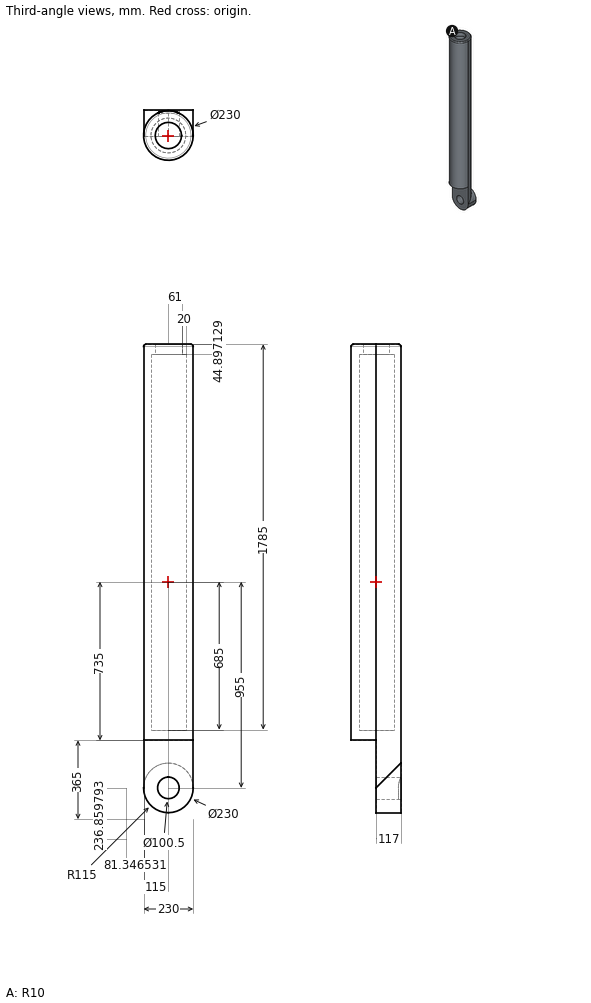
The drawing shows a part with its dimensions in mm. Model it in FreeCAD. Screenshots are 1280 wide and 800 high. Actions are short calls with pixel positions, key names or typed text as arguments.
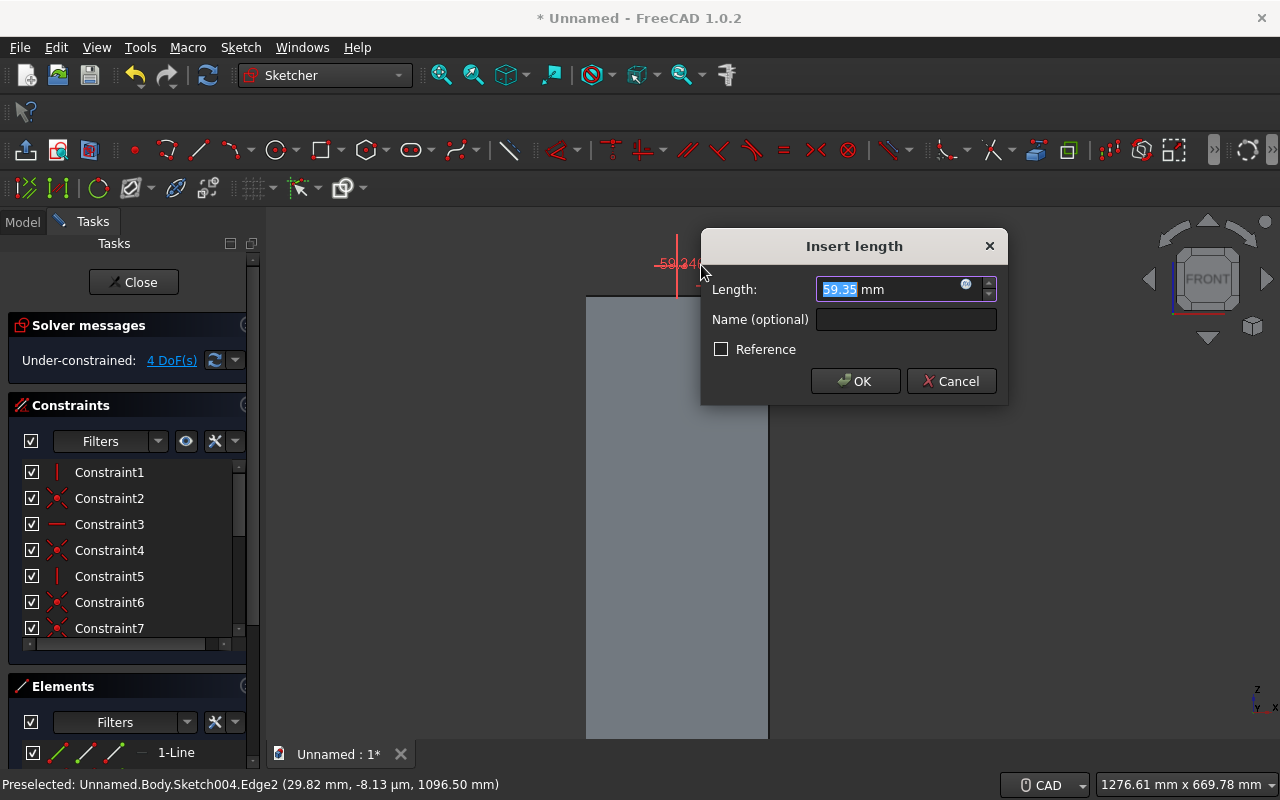
text(61)
key(Return)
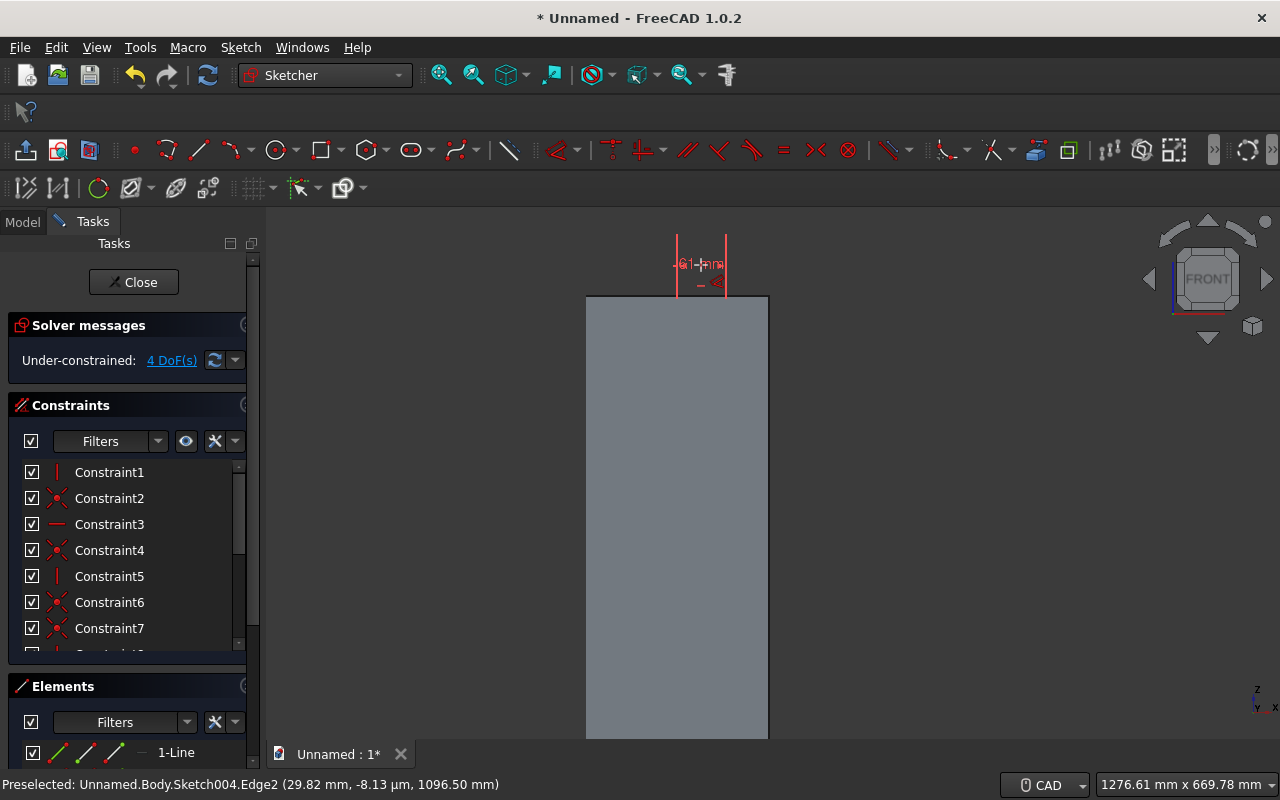
scroll(734, 336, up, 5)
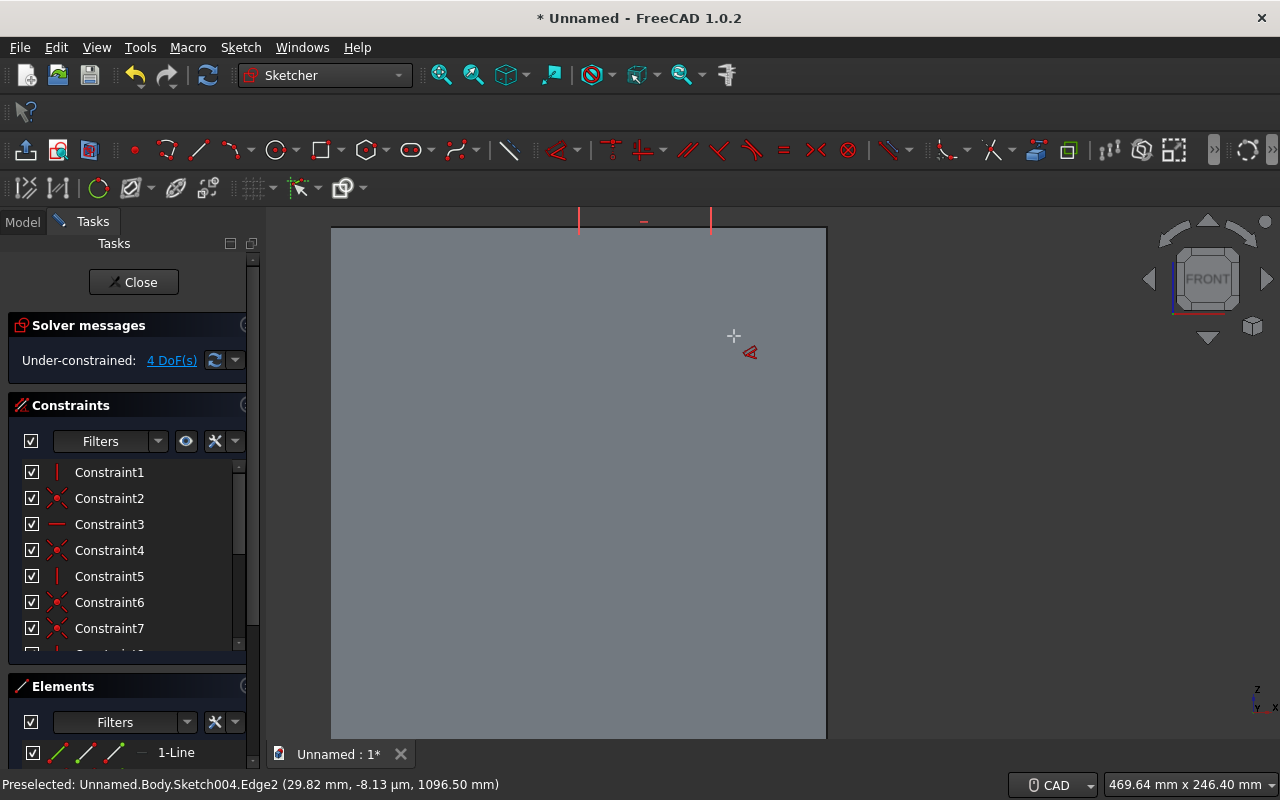
click(732, 335)
click(732, 301)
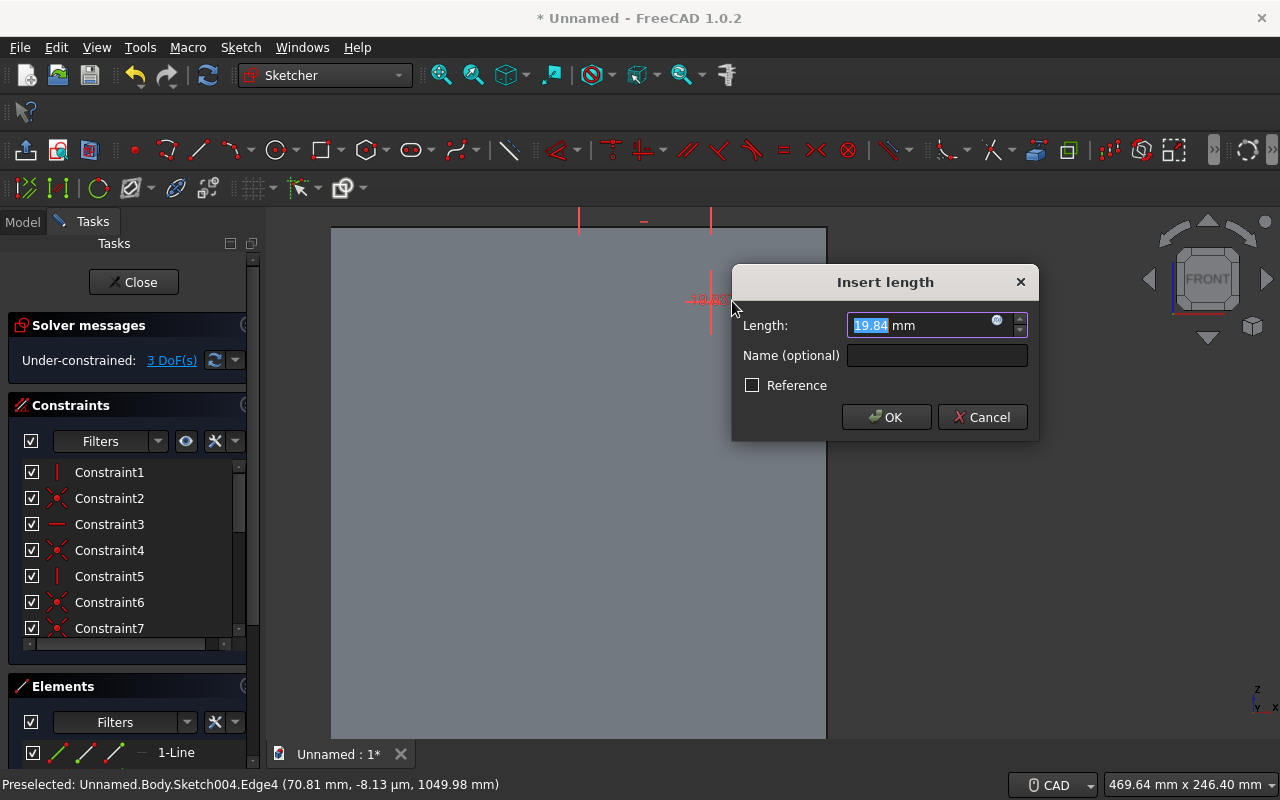
text(20)
key(Return)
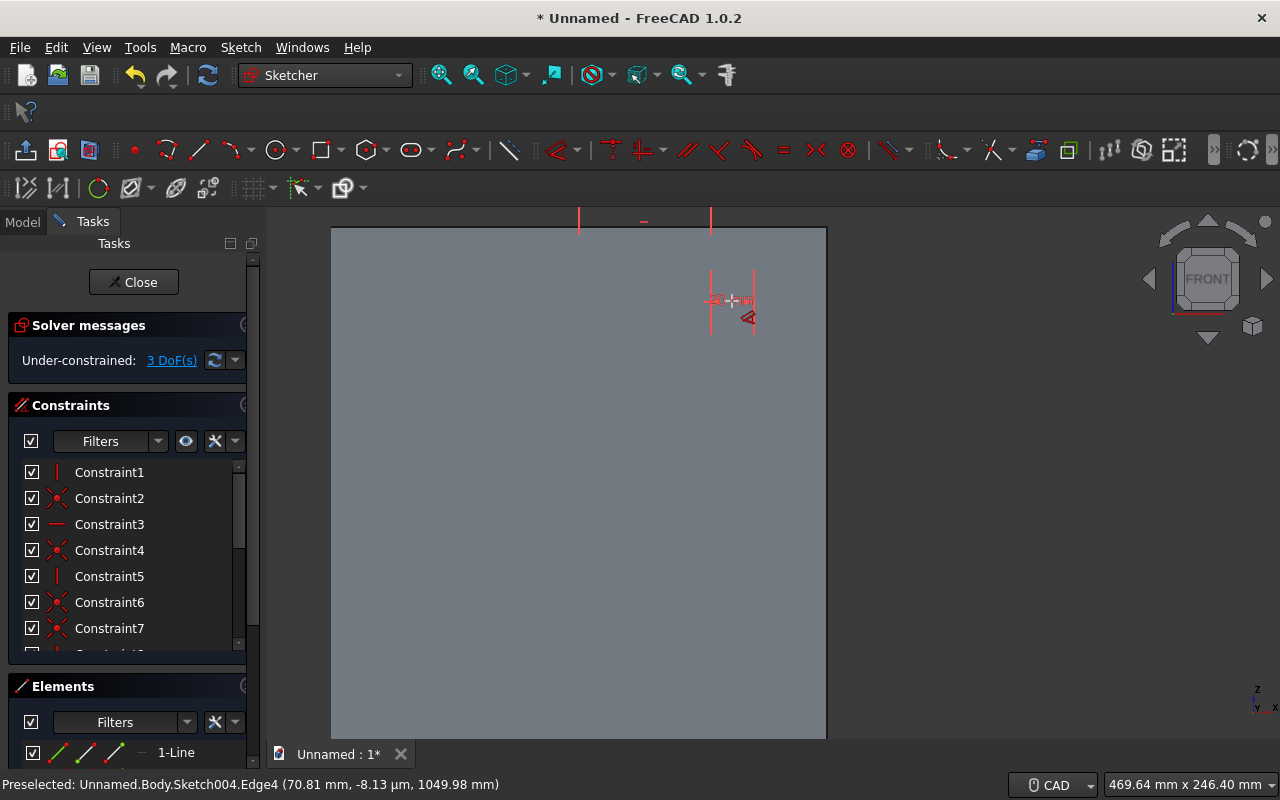
scroll(708, 305, down, 12)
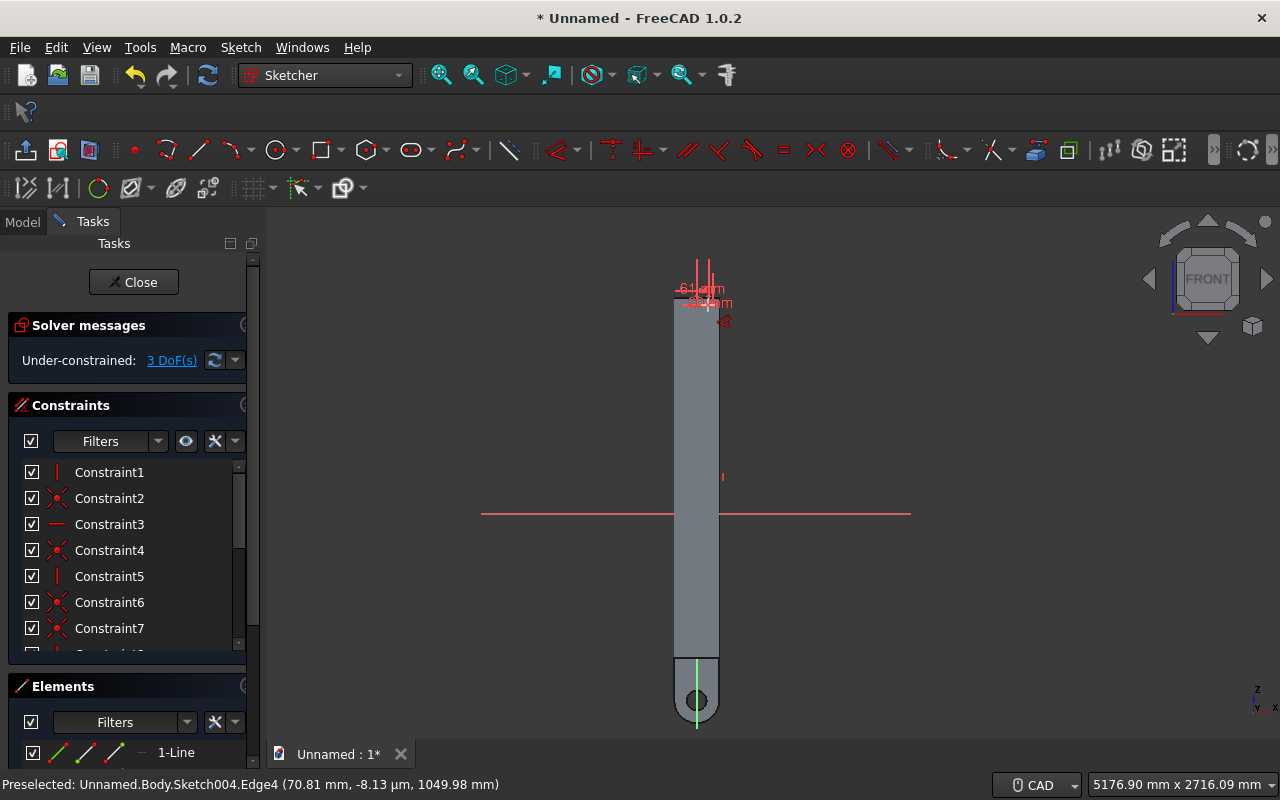
click(697, 544)
click(663, 474)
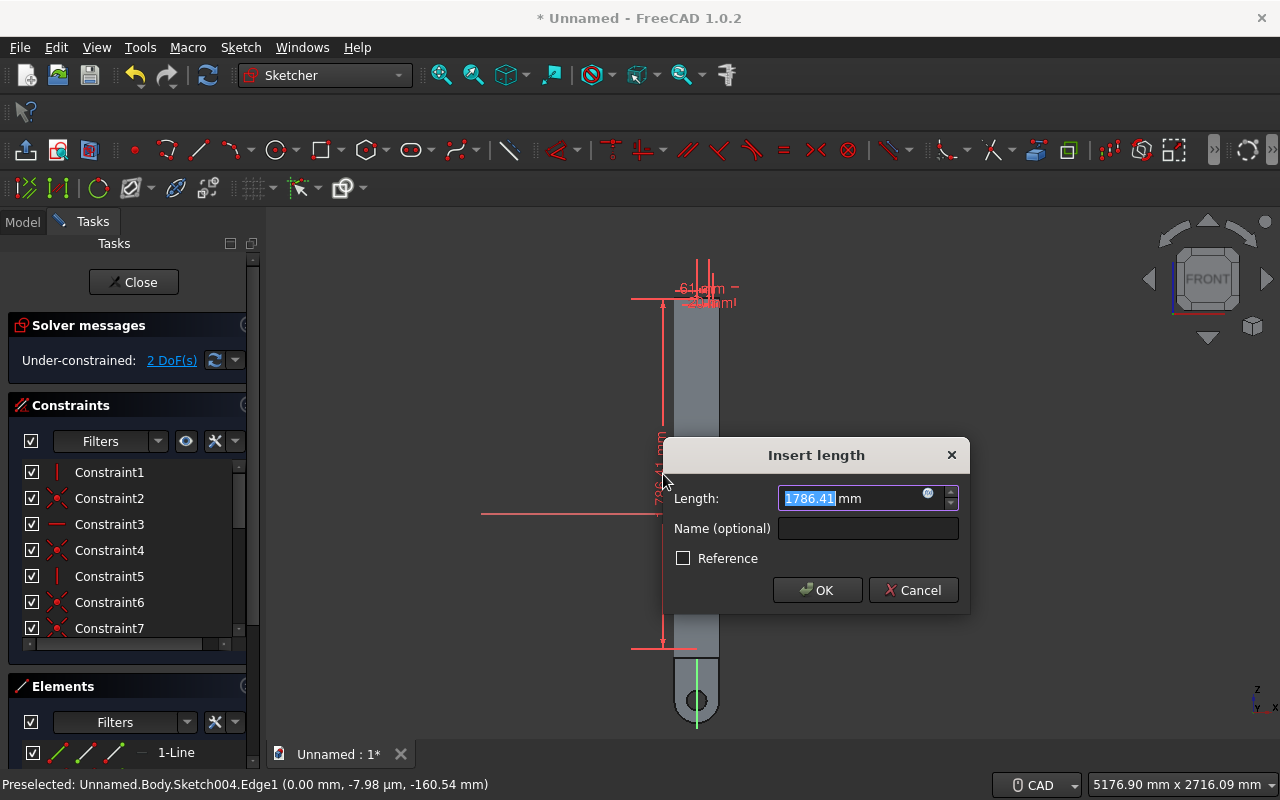
text(1785)
key(Return)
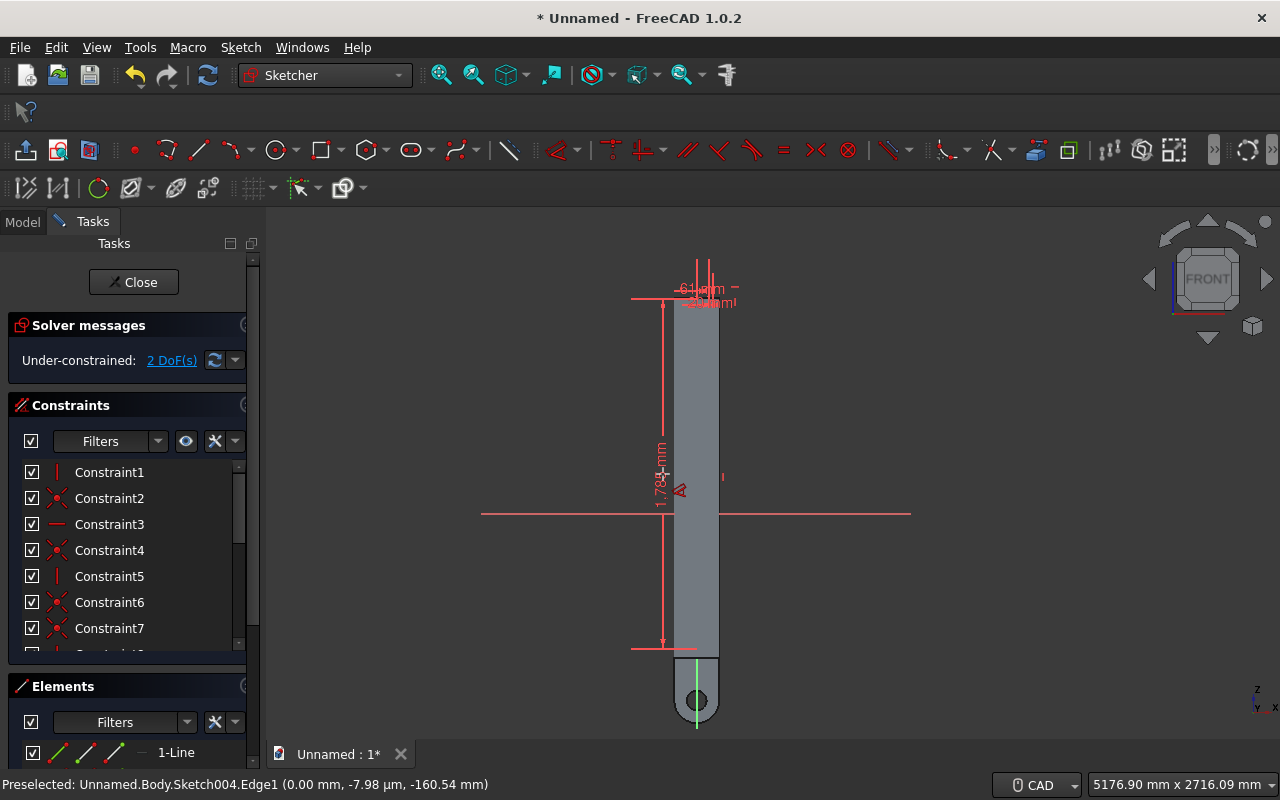
click(697, 649)
click(663, 581)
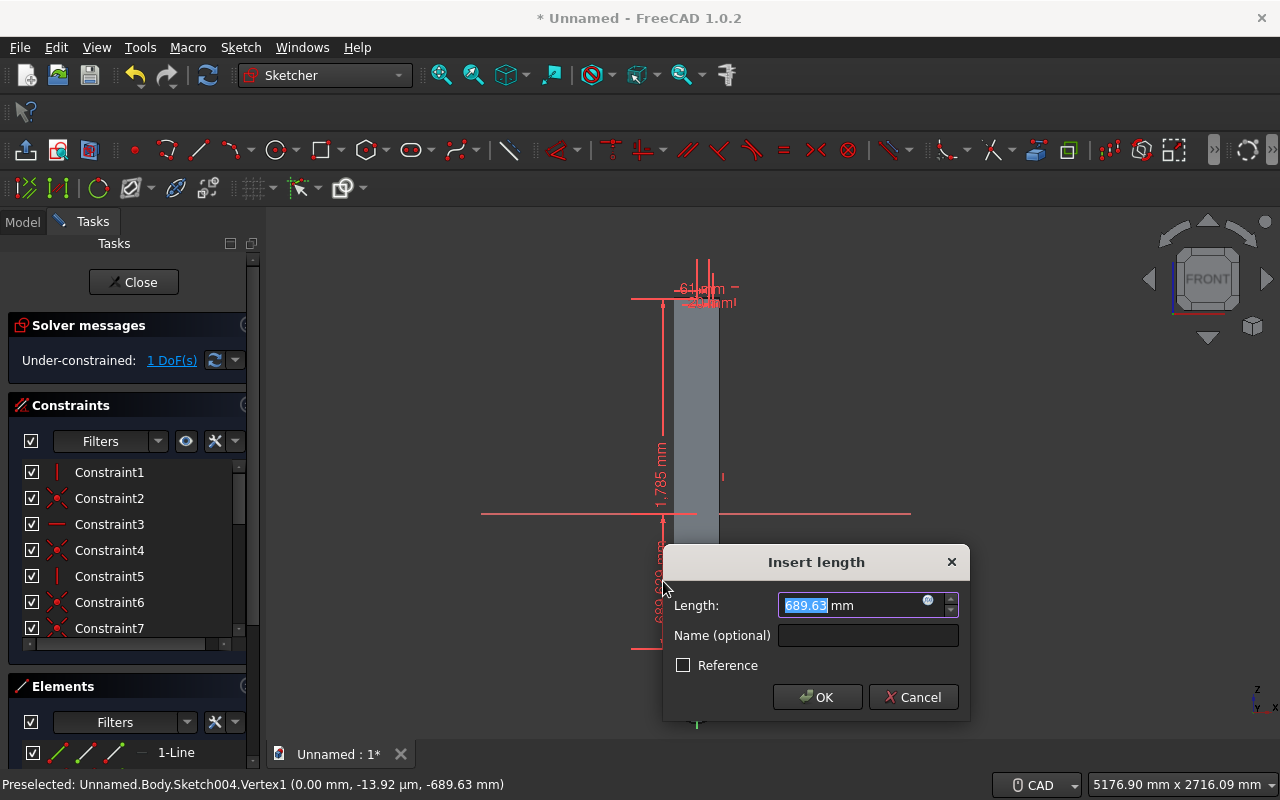
text(685)
key(Return)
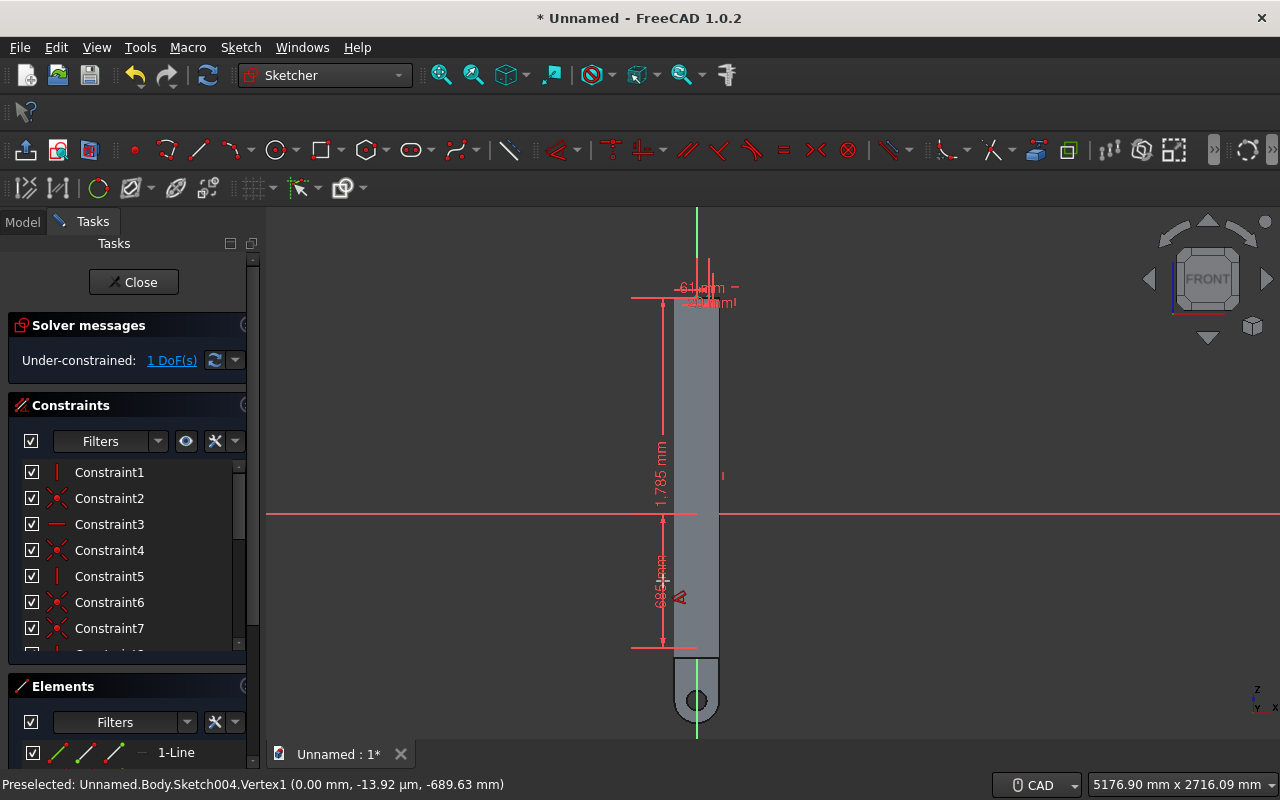
scroll(709, 303, up, 8)